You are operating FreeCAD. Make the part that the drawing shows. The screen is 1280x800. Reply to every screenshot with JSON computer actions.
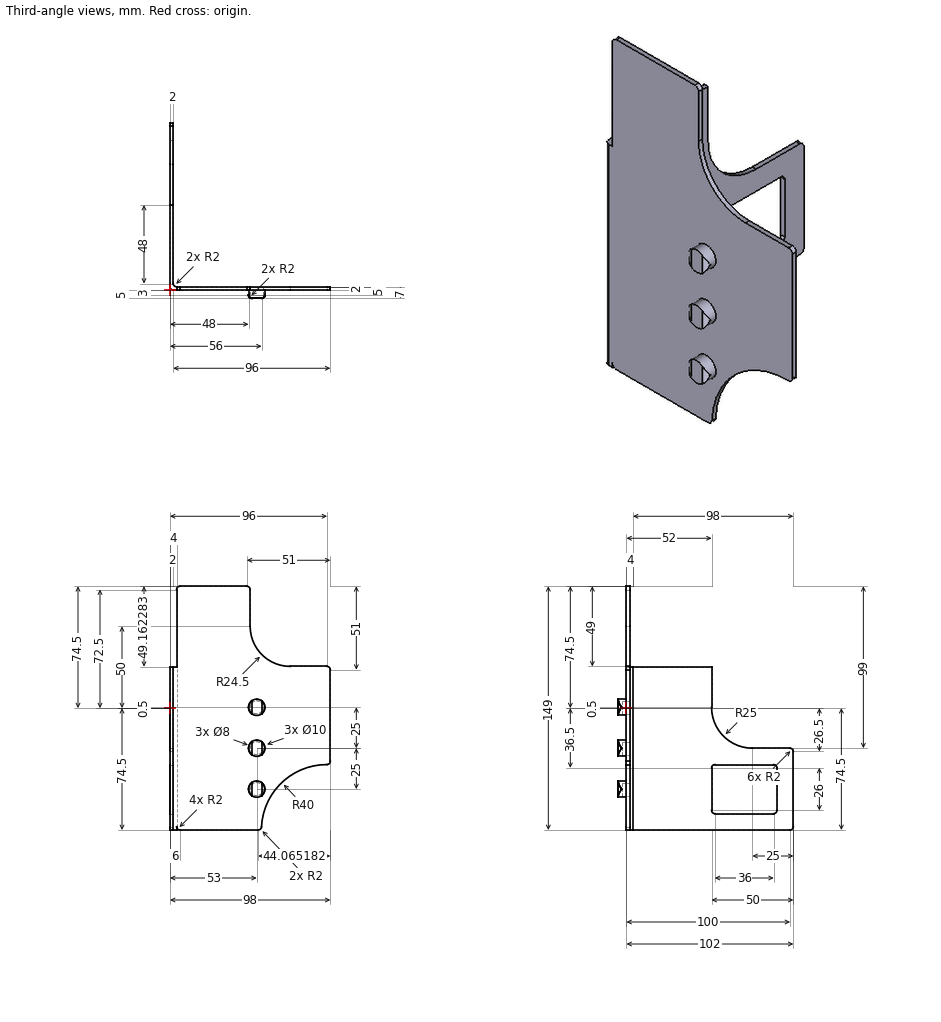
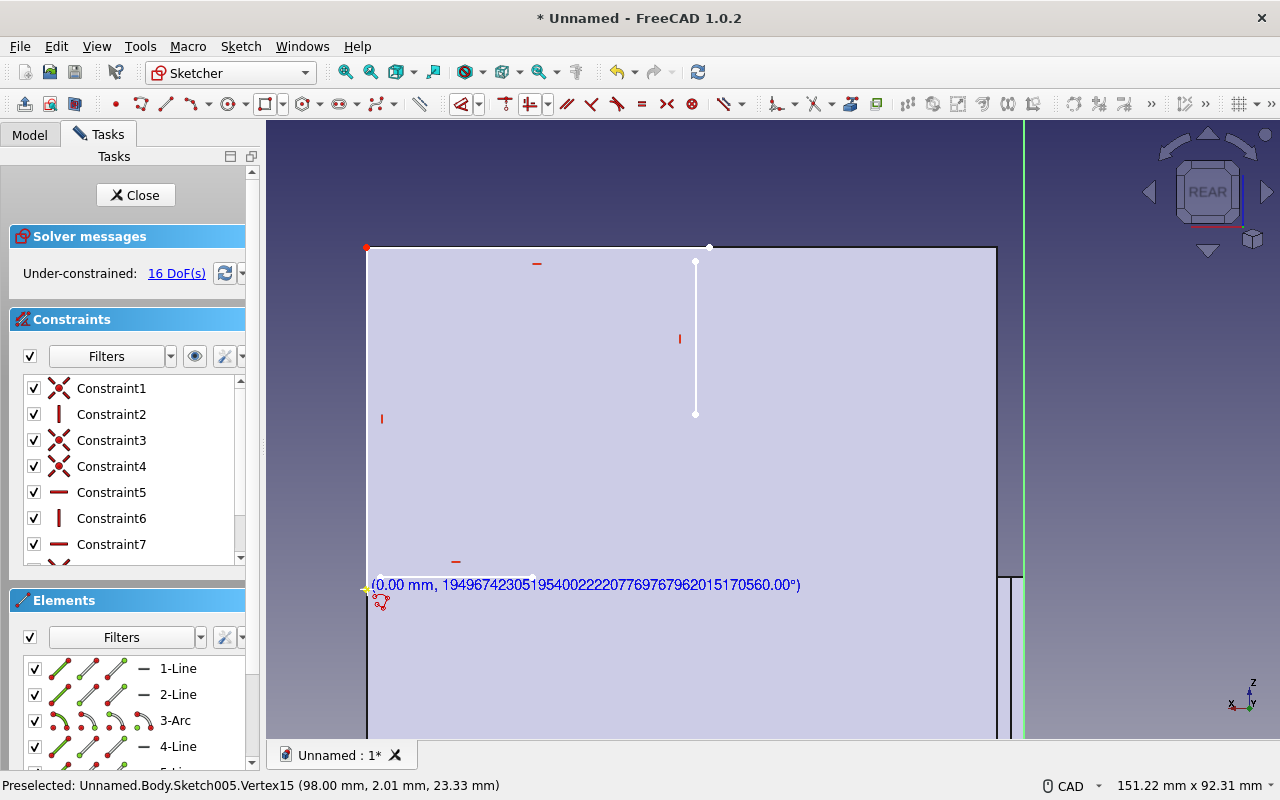
{"action": "key", "text": "g 3 a"}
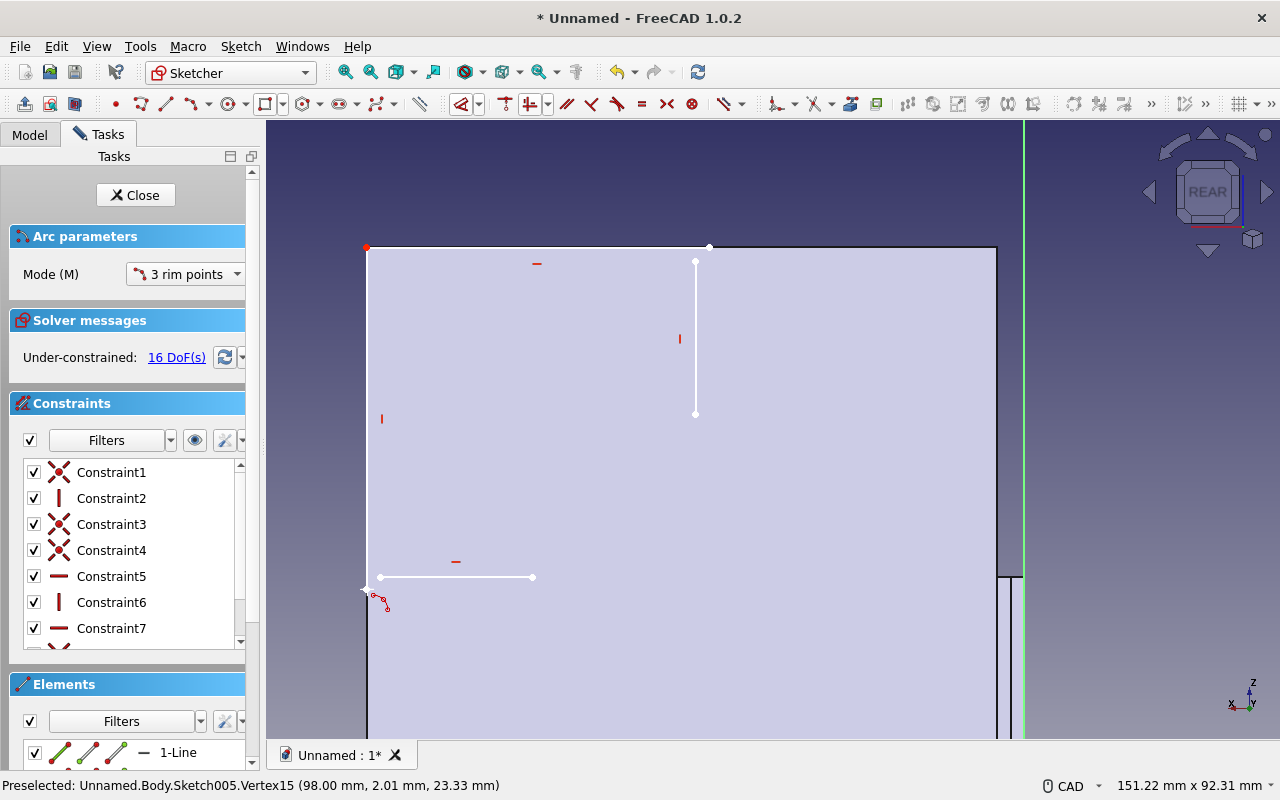
{"action": "left_click", "coordinate": [533, 577]}
{"action": "left_click", "coordinate": [696, 414]}
{"action": "left_click", "coordinate": [647, 527]}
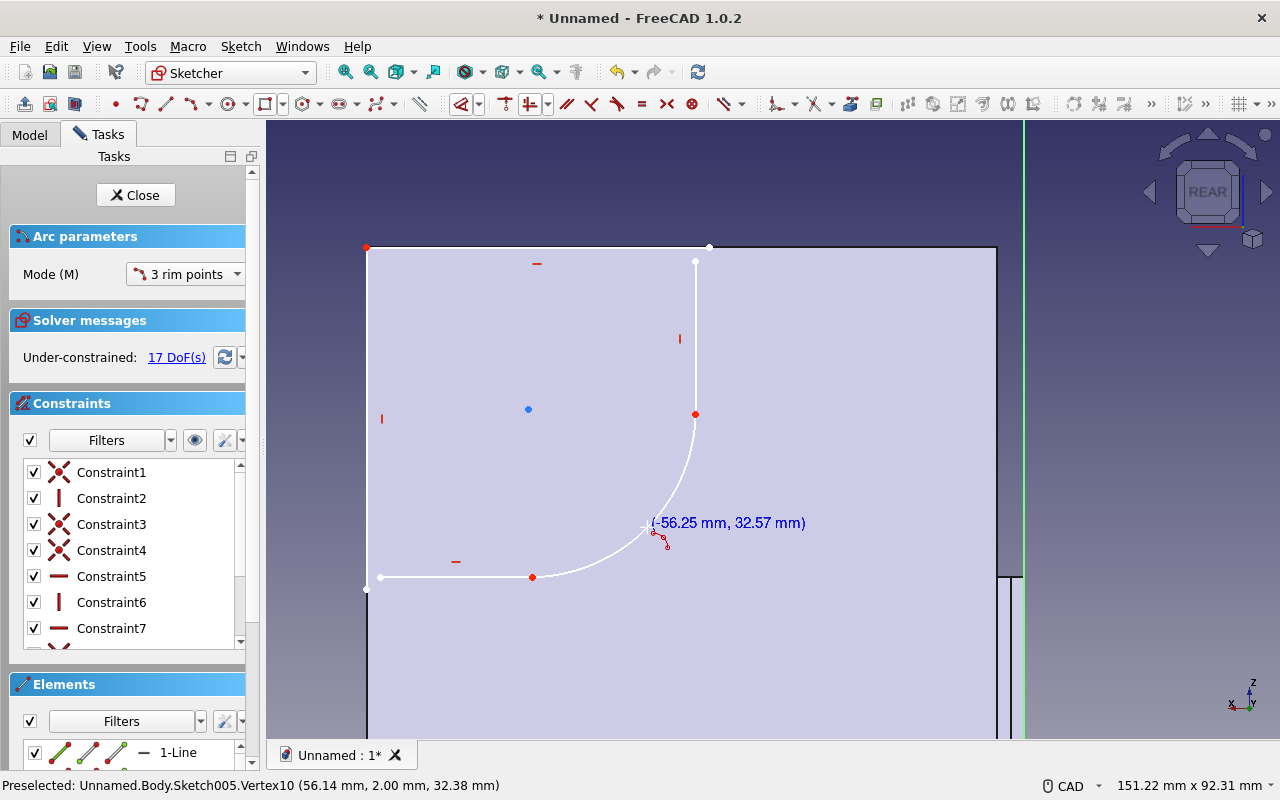
{"action": "left_click", "coordinate": [696, 262]}
{"action": "left_click", "coordinate": [709, 248]}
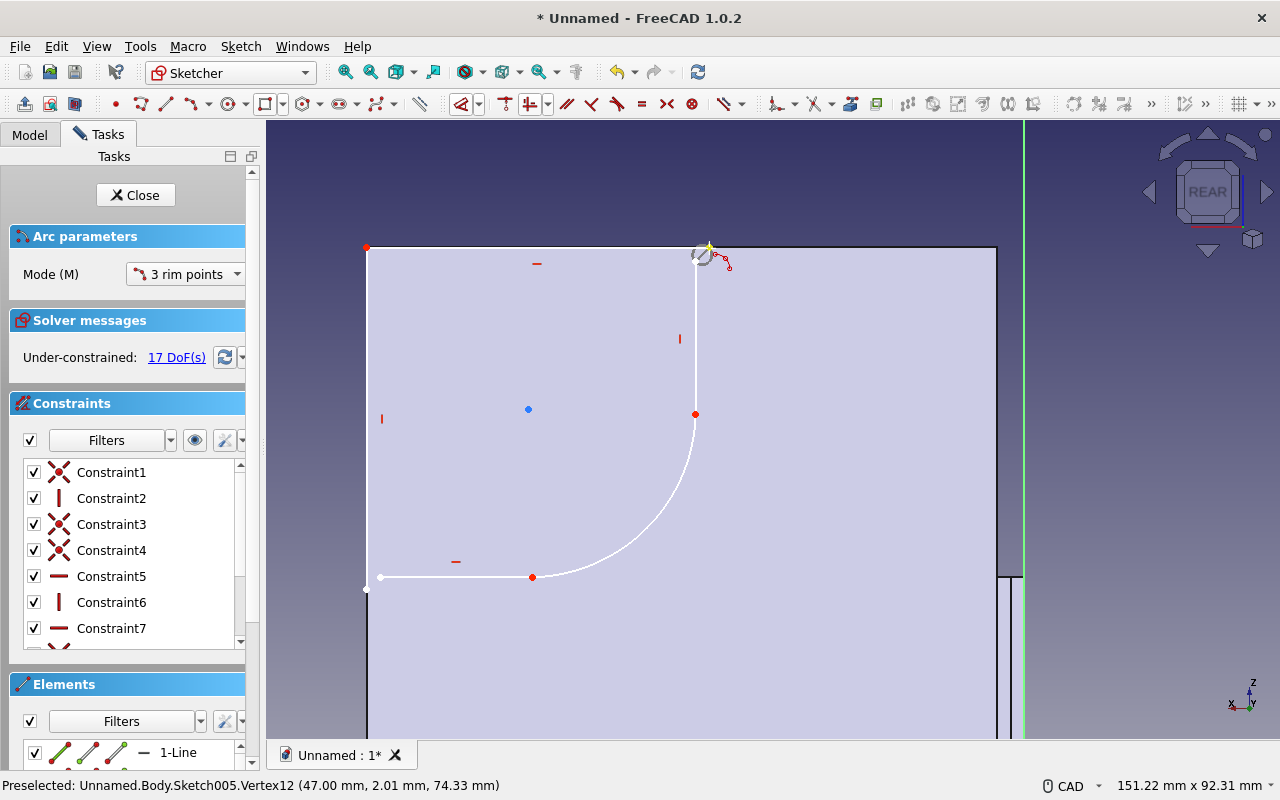
{"action": "scroll", "coordinate": [700, 251], "scroll_direction": "up", "scroll_amount": 7}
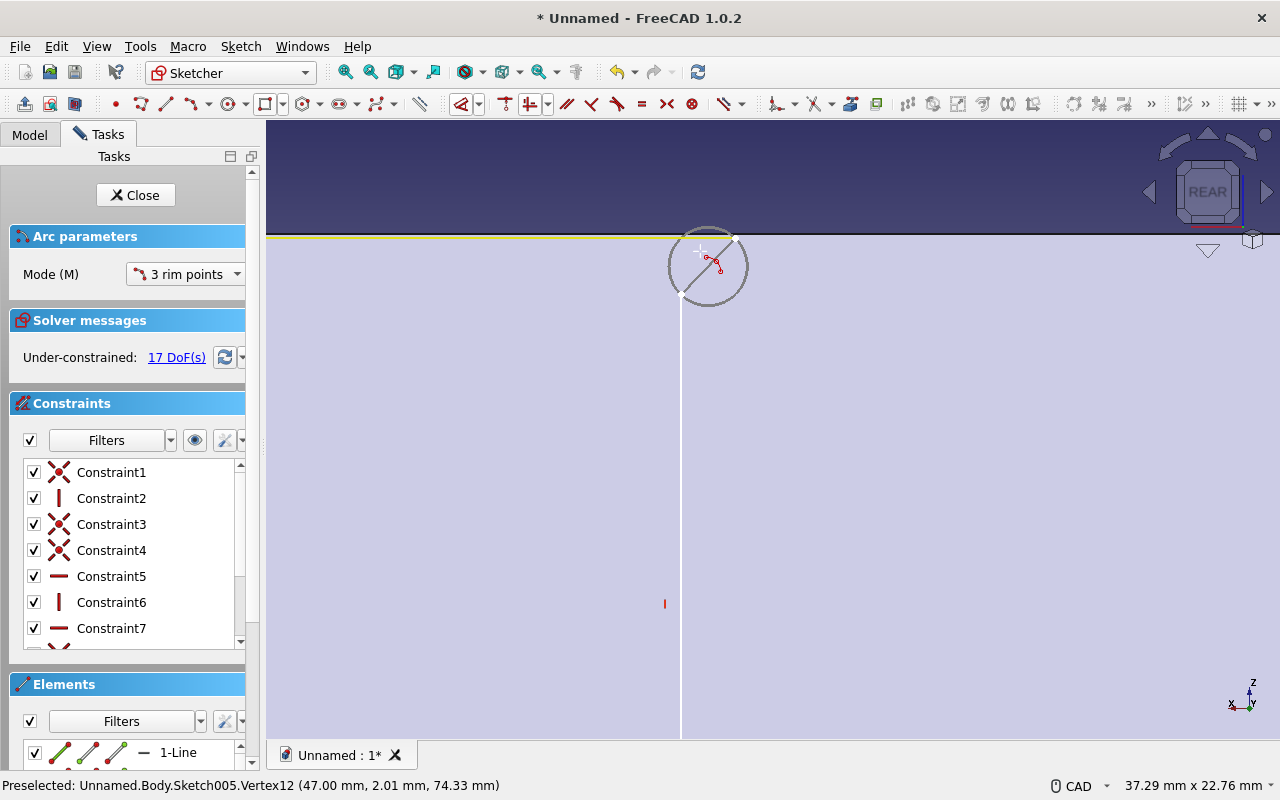
{"action": "left_click", "coordinate": [697, 250]}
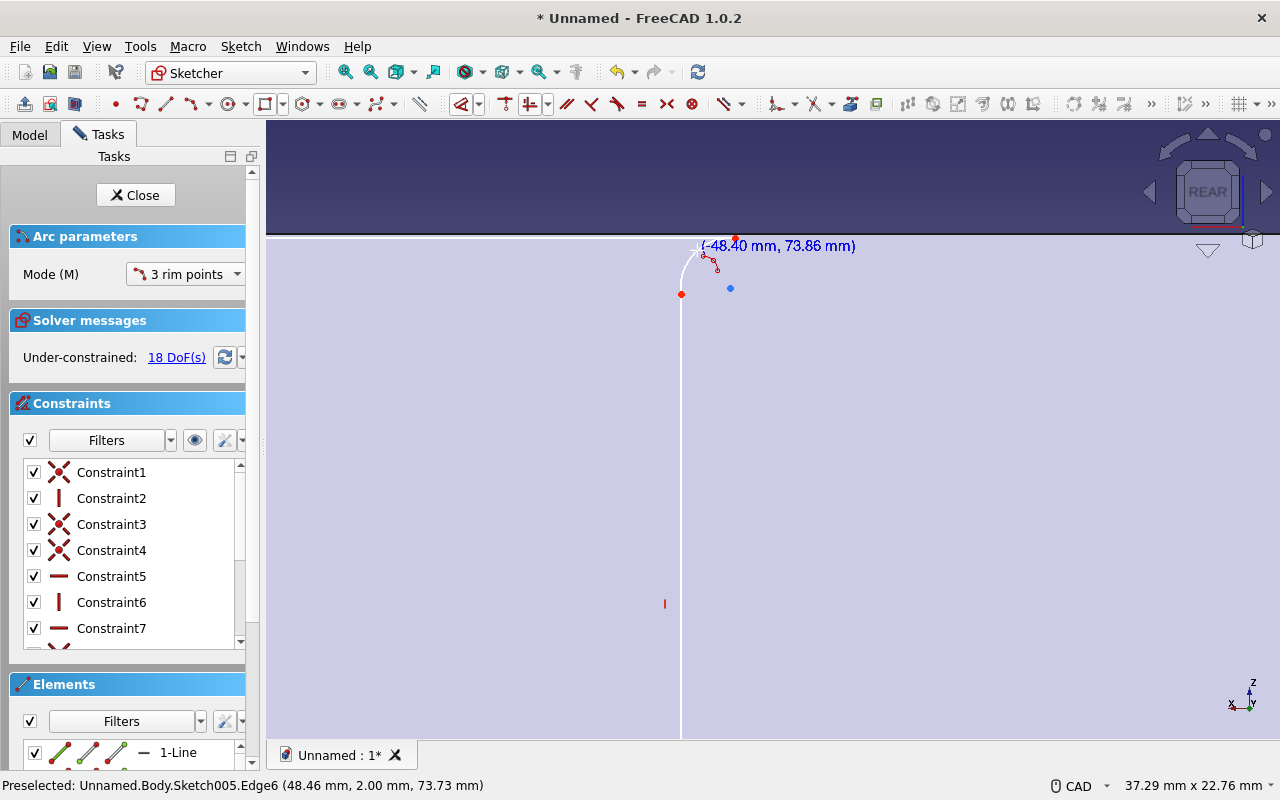
{"action": "scroll", "coordinate": [707, 247], "scroll_direction": "down", "scroll_amount": 12}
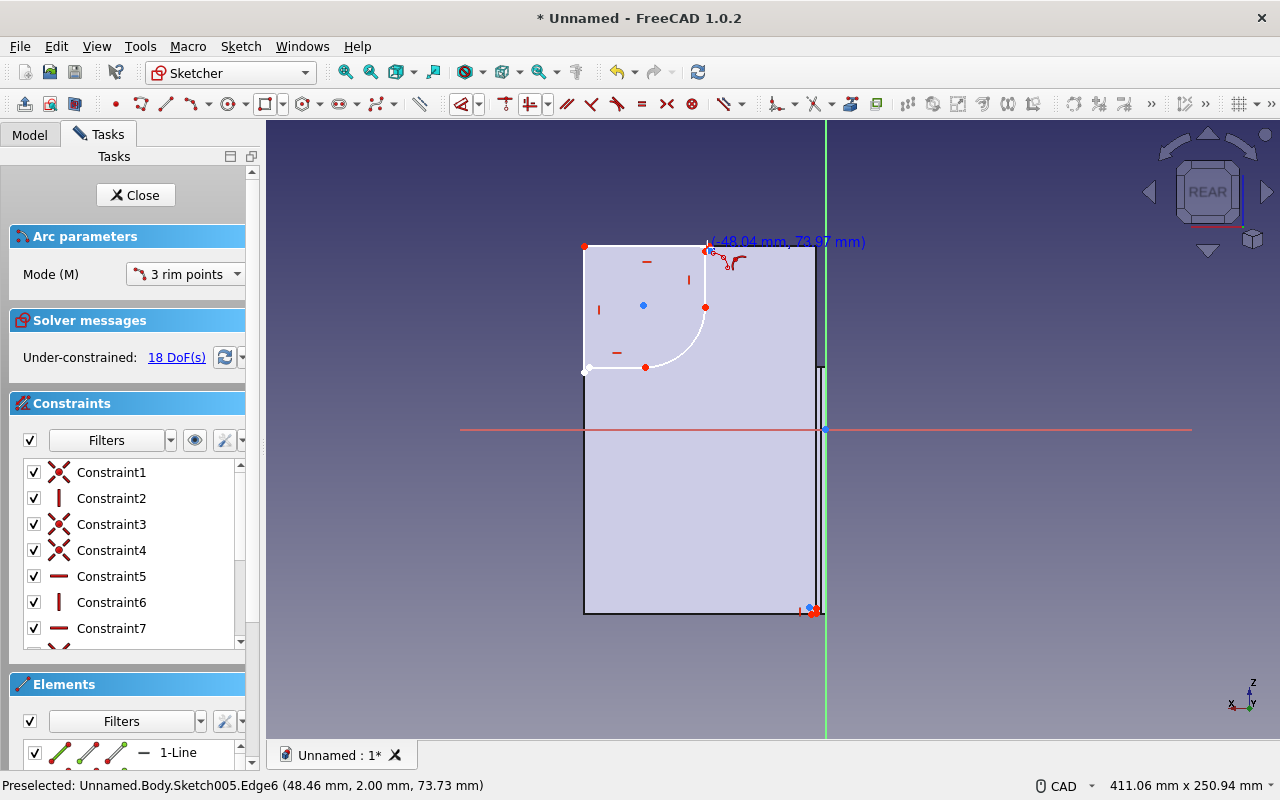
{"action": "scroll", "coordinate": [584, 372], "scroll_direction": "up", "scroll_amount": 5}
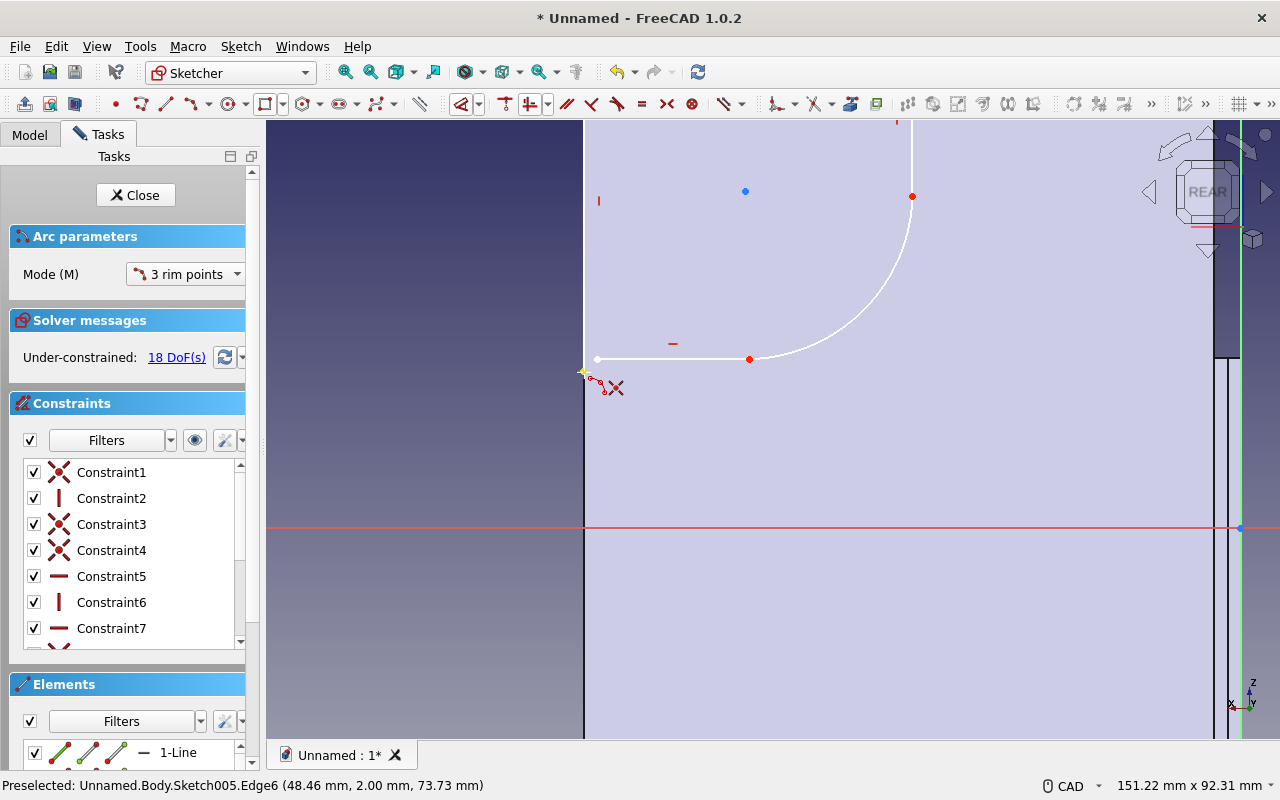
{"action": "left_click", "coordinate": [584, 372]}
{"action": "left_click", "coordinate": [597, 359]}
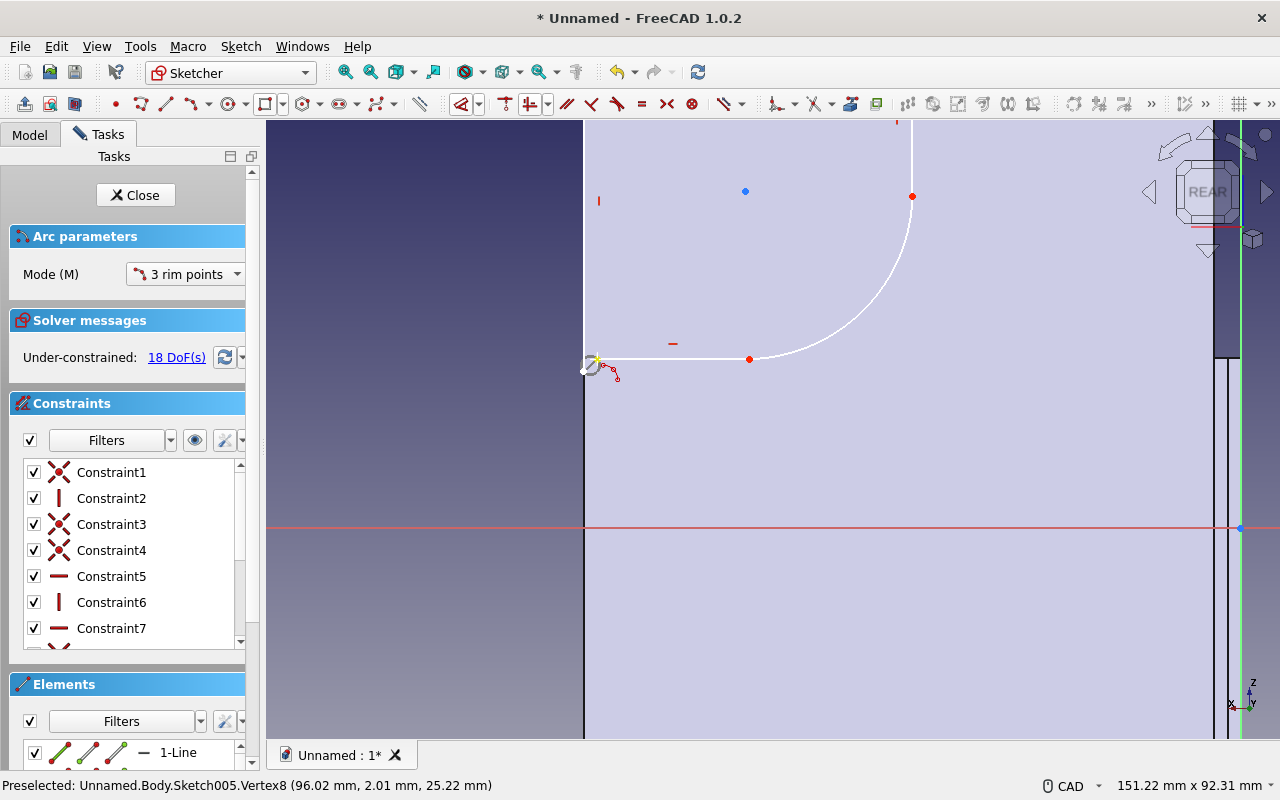
{"action": "scroll", "coordinate": [588, 361], "scroll_direction": "up", "scroll_amount": 7}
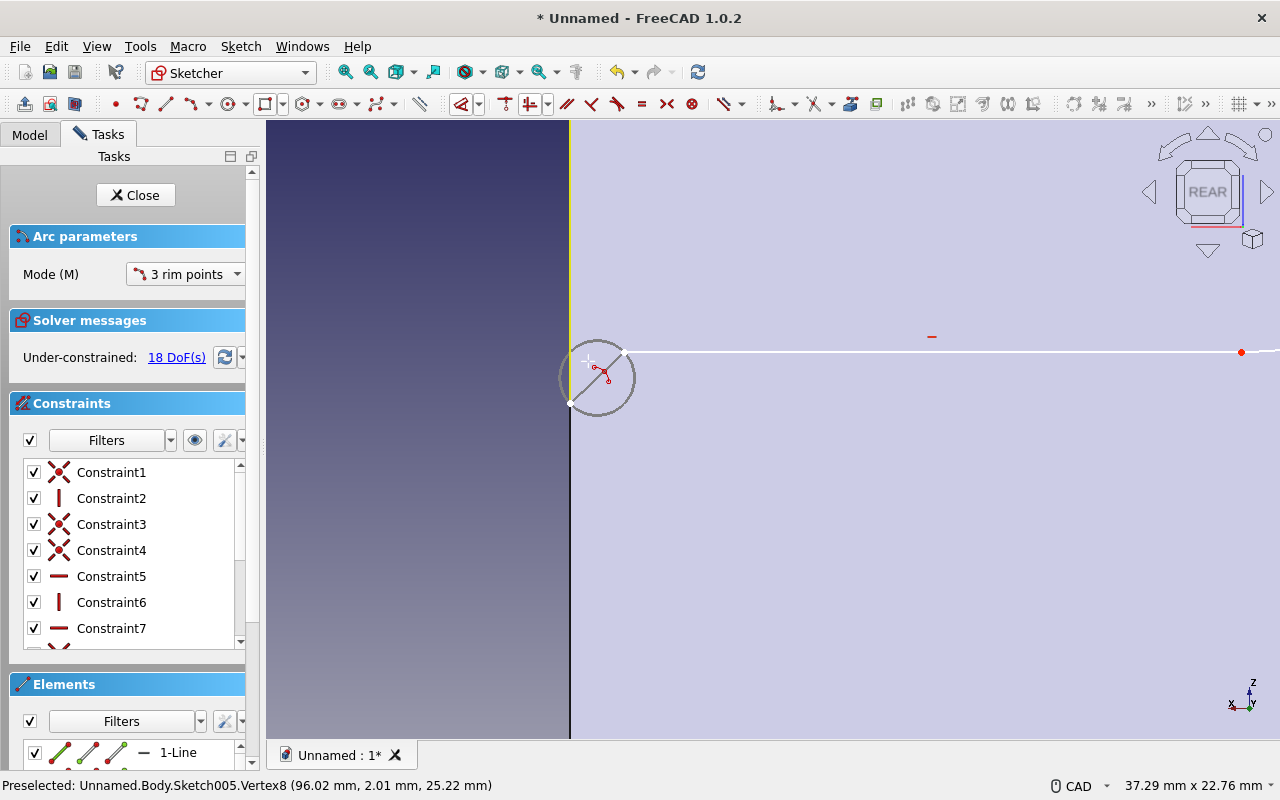
{"action": "left_click", "coordinate": [586, 361]}